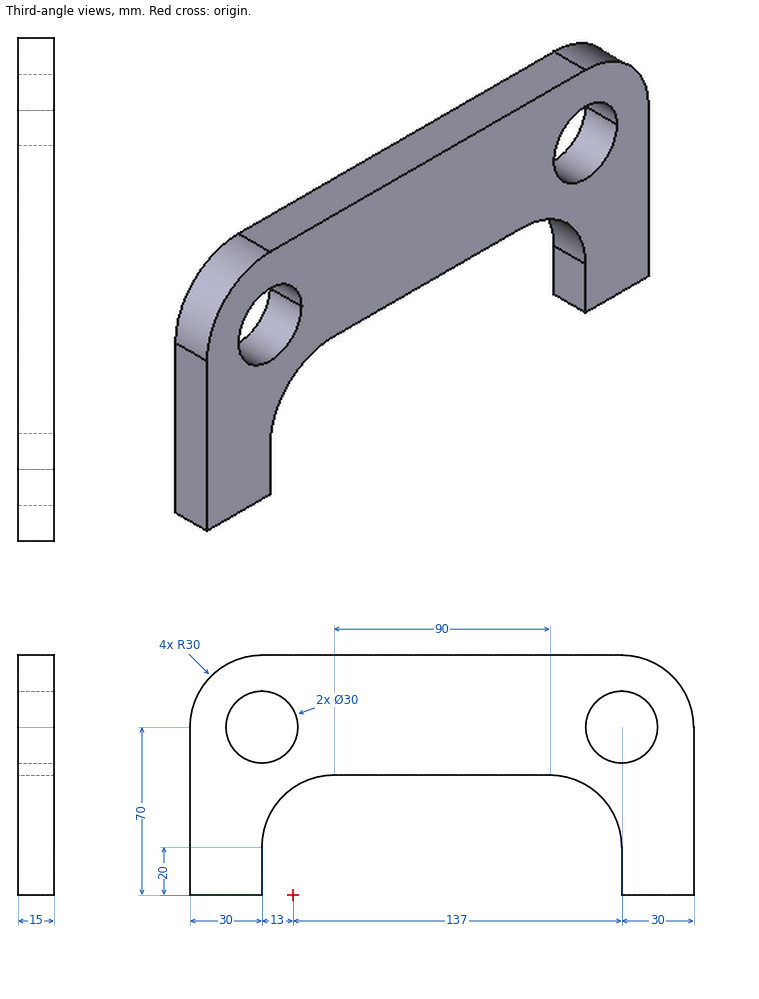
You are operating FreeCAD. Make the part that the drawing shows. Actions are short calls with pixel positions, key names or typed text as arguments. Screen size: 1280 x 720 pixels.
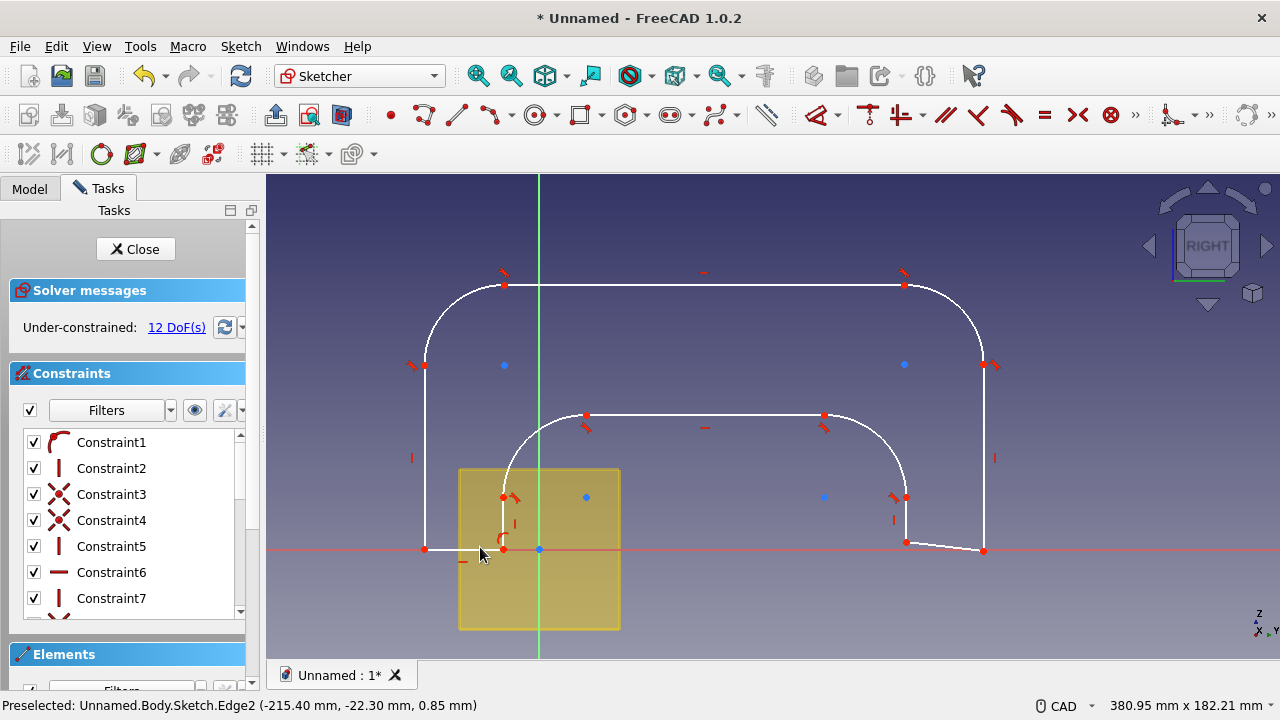
click(960, 548)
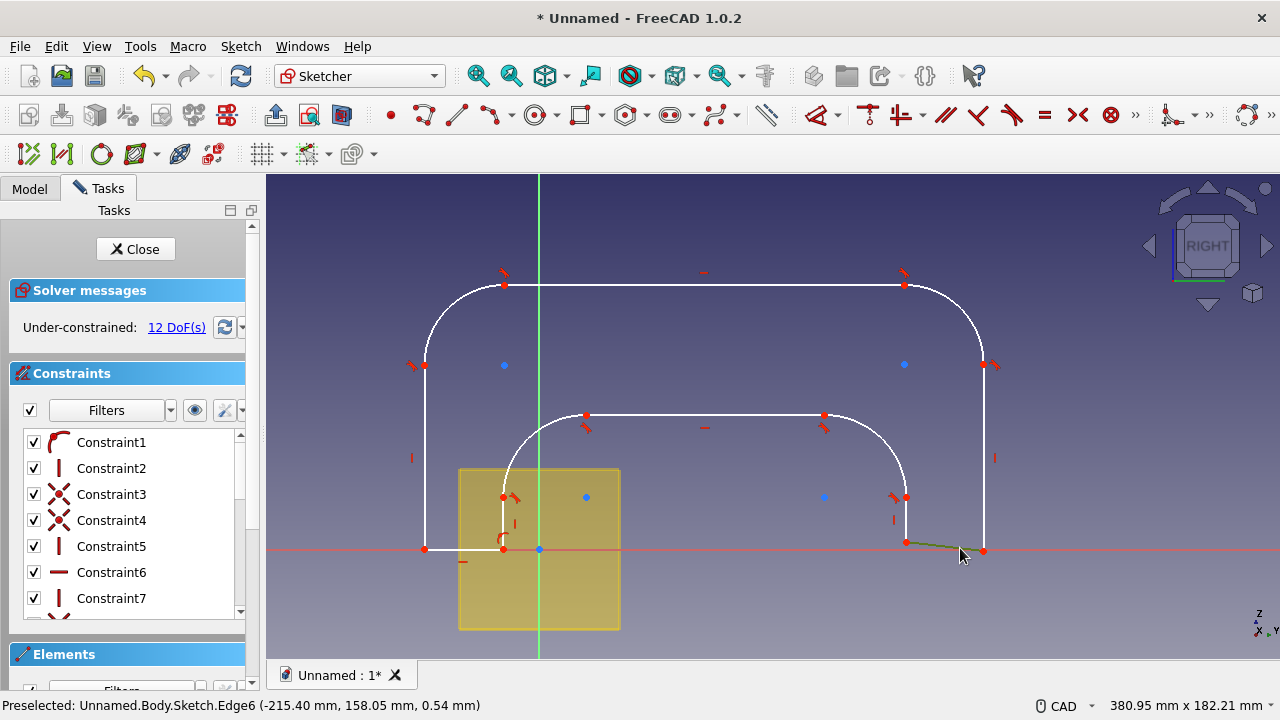
key(h)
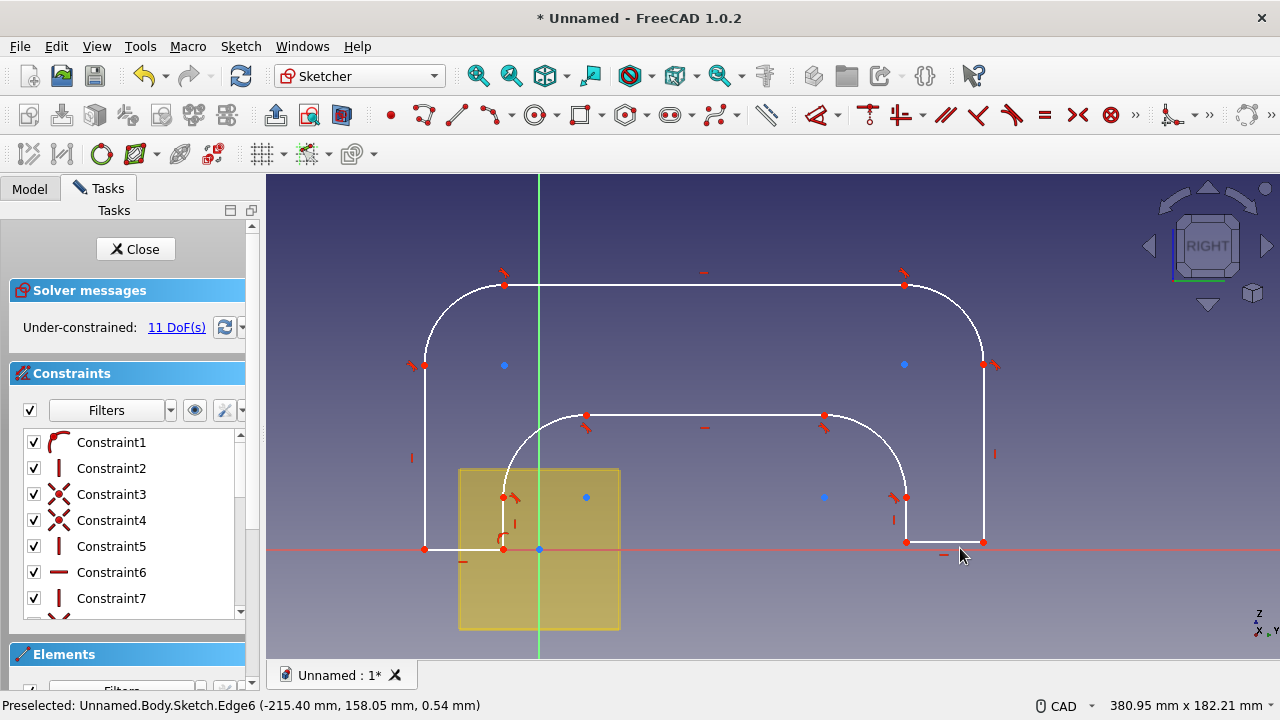
click(468, 294)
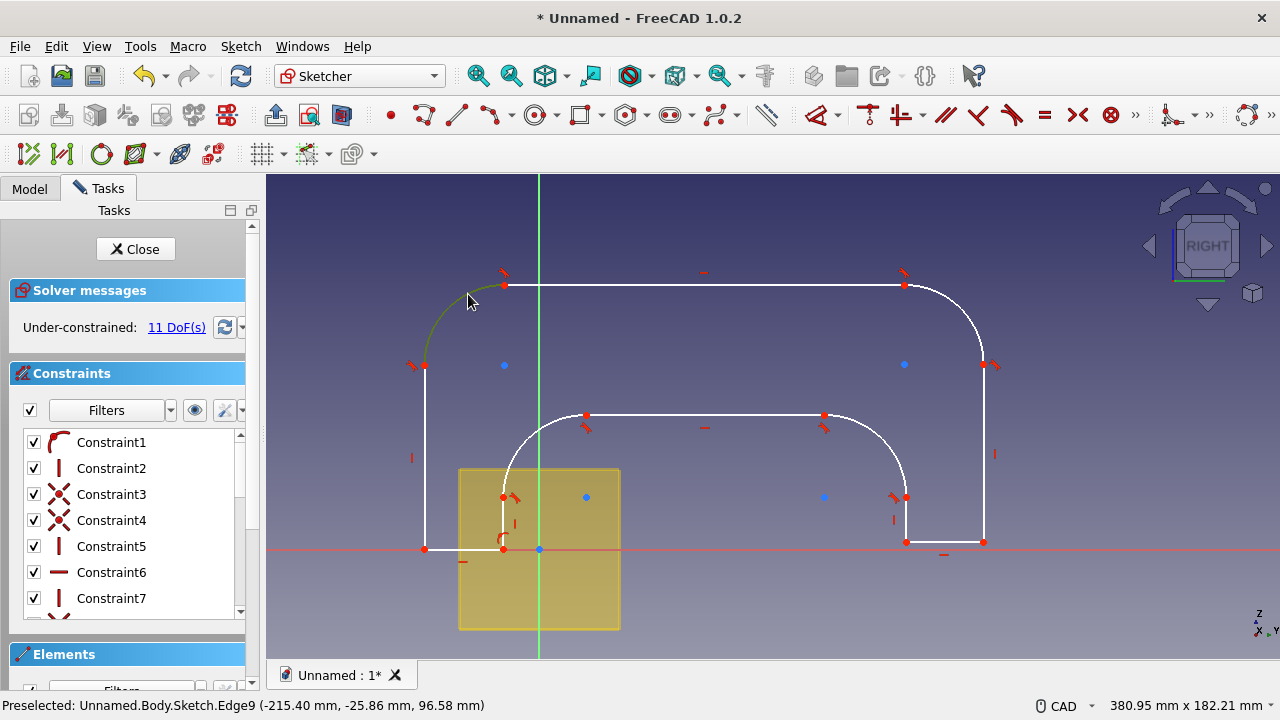
click(975, 328)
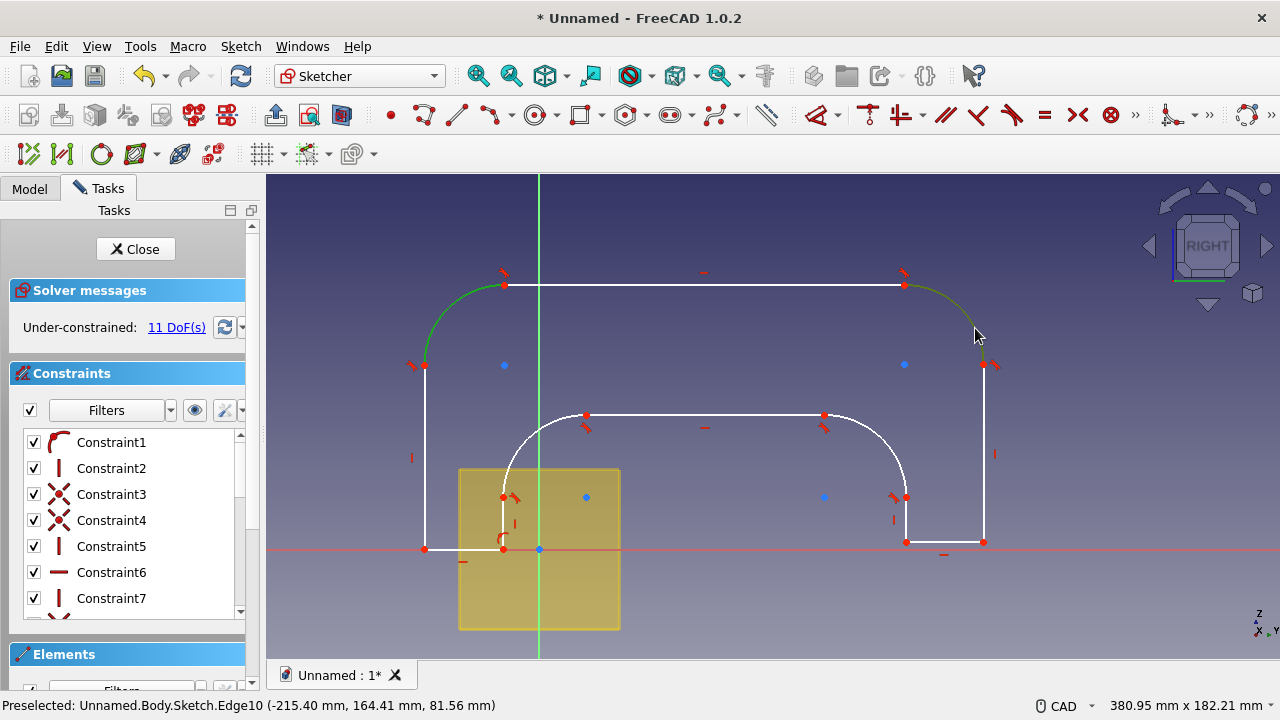
click(897, 460)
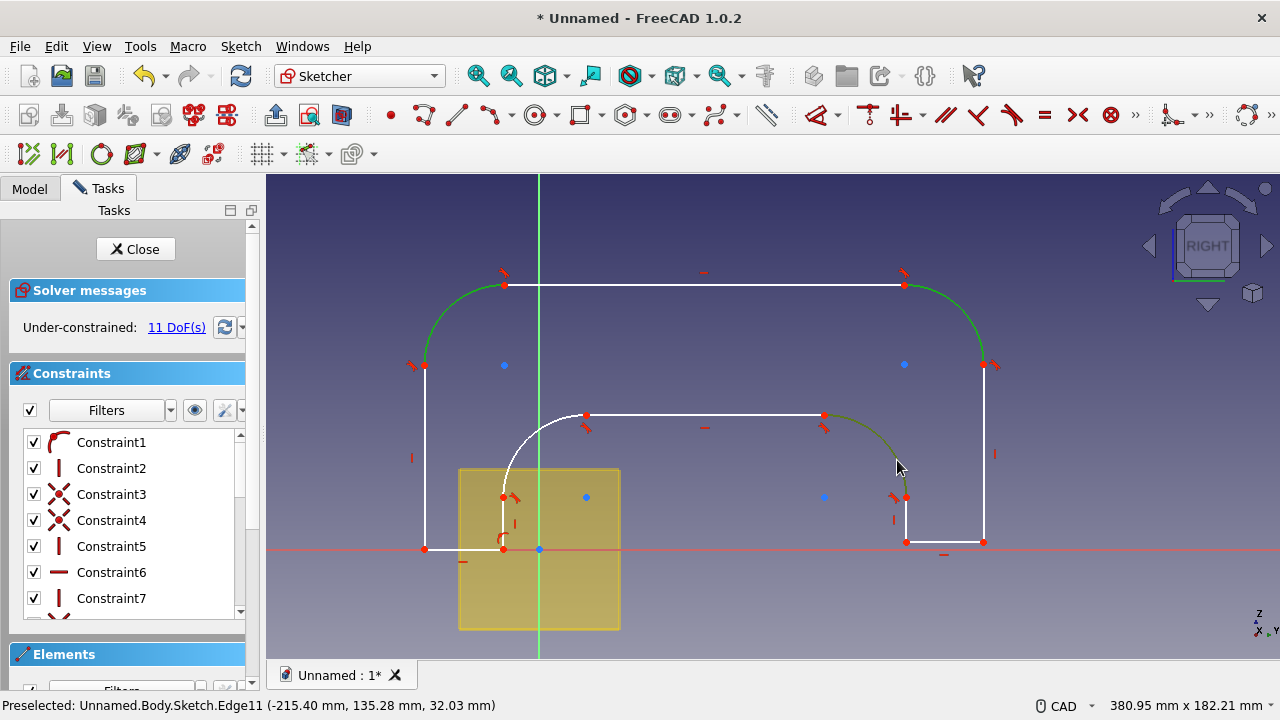
scroll(548, 424, up, 3)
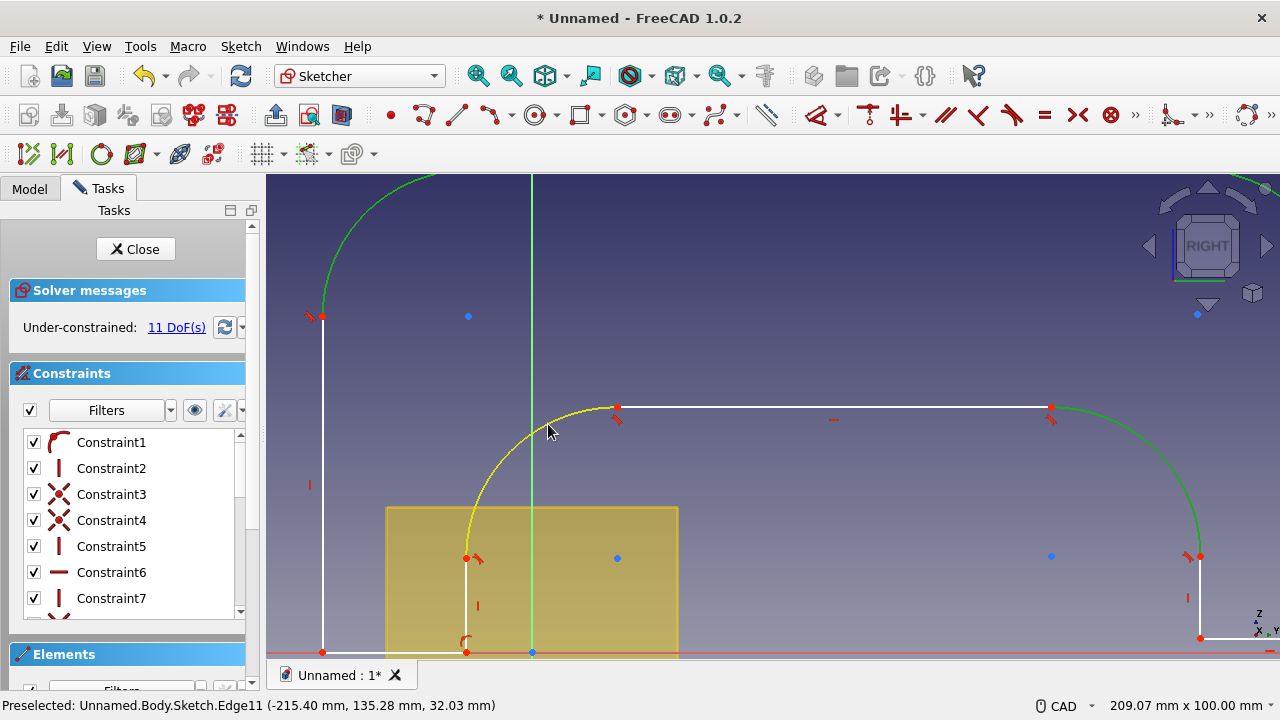
click(549, 424)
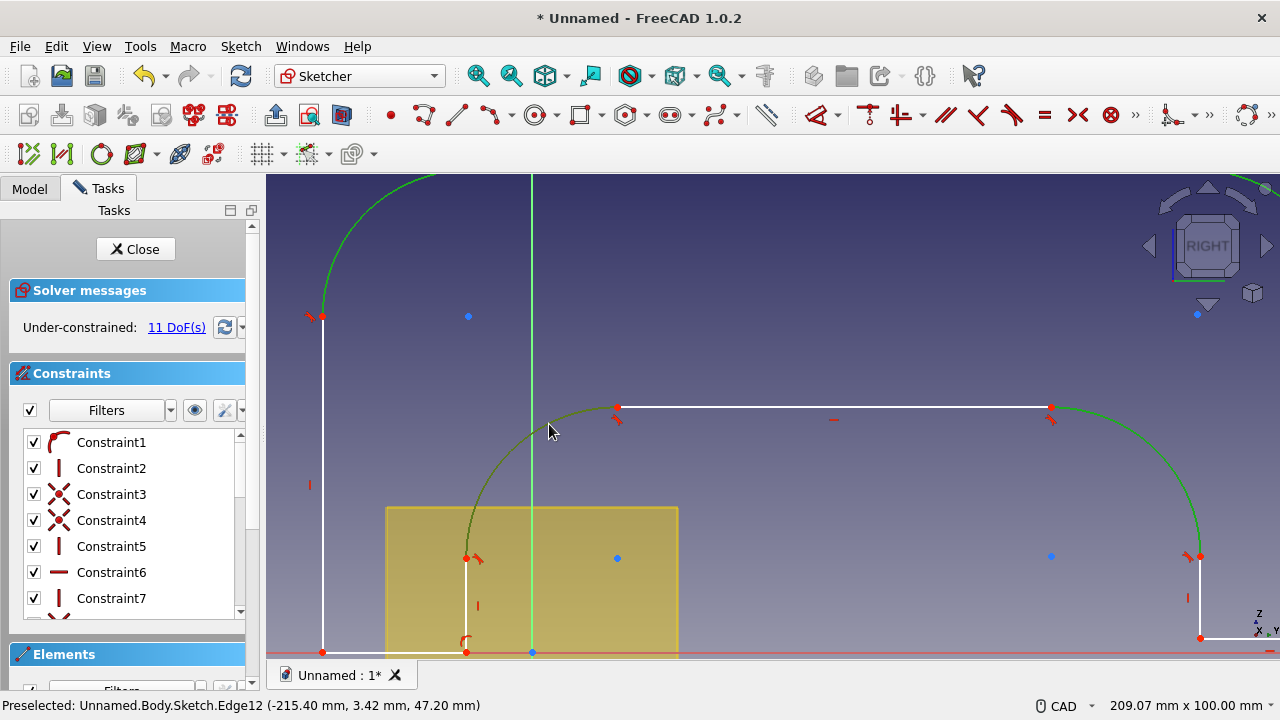
key(e)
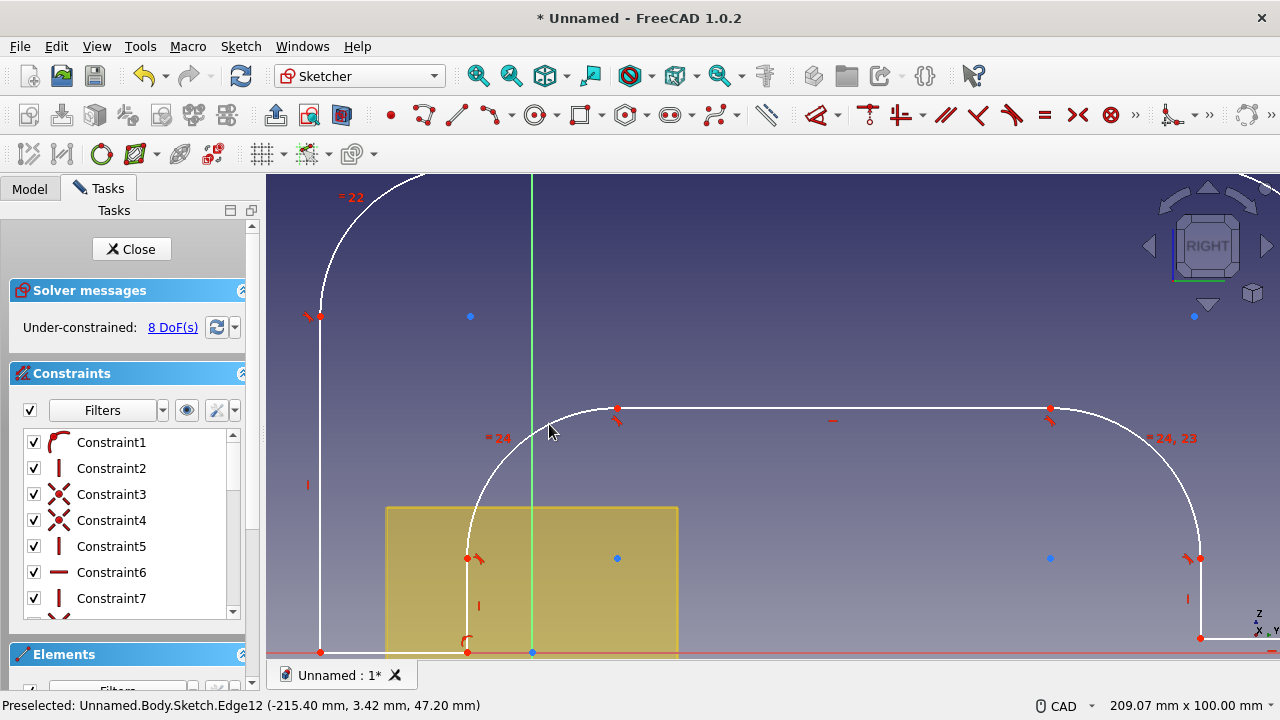
key(d)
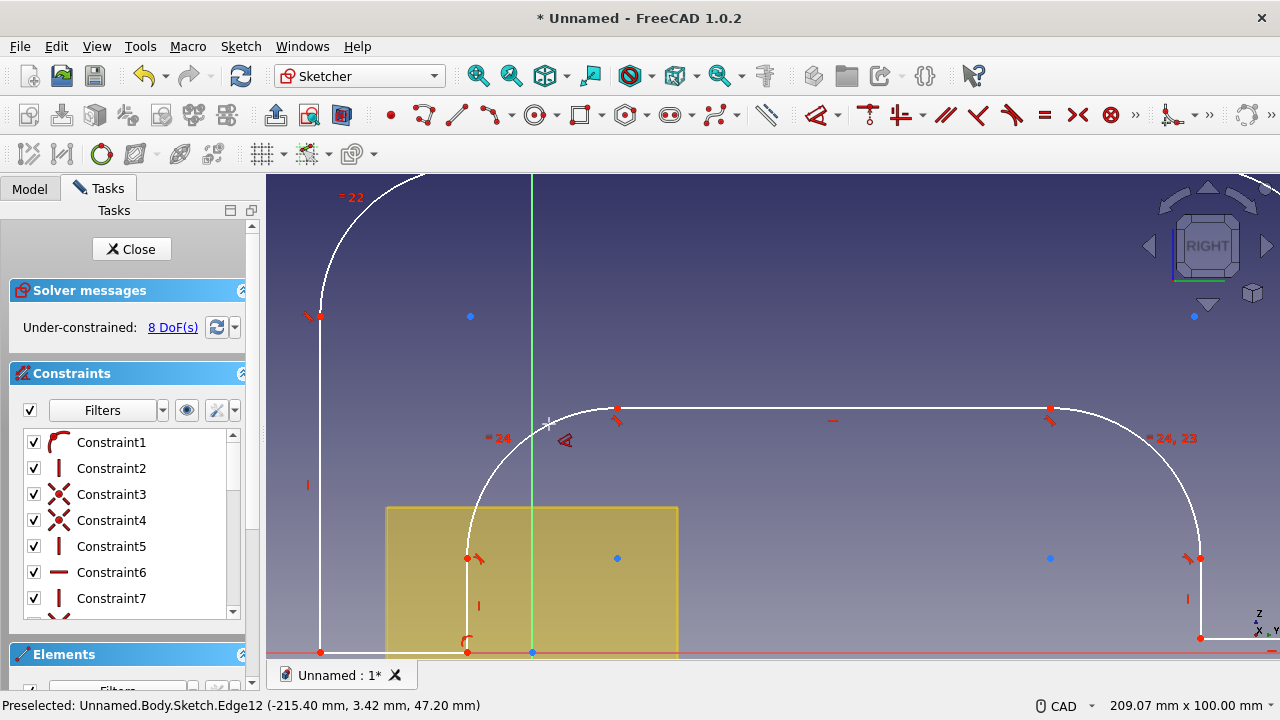
click(337, 249)
click(308, 234)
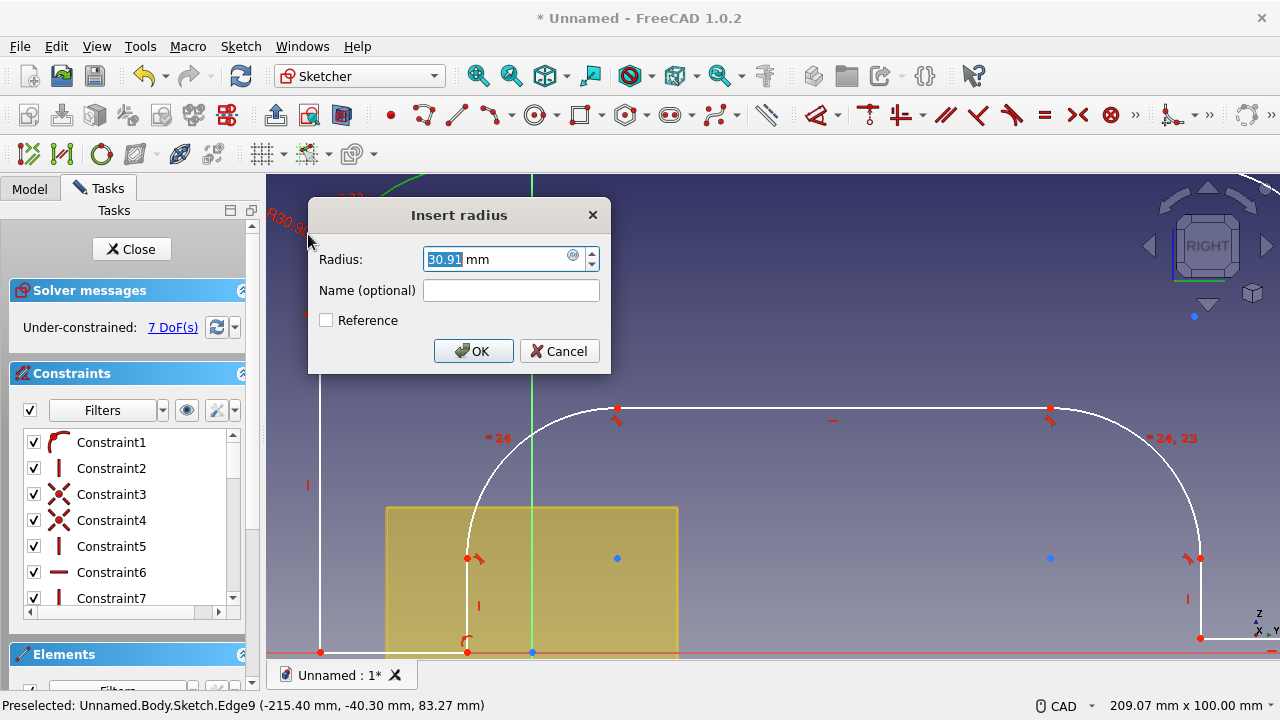
text(30)
key(Return)
key(Escape)